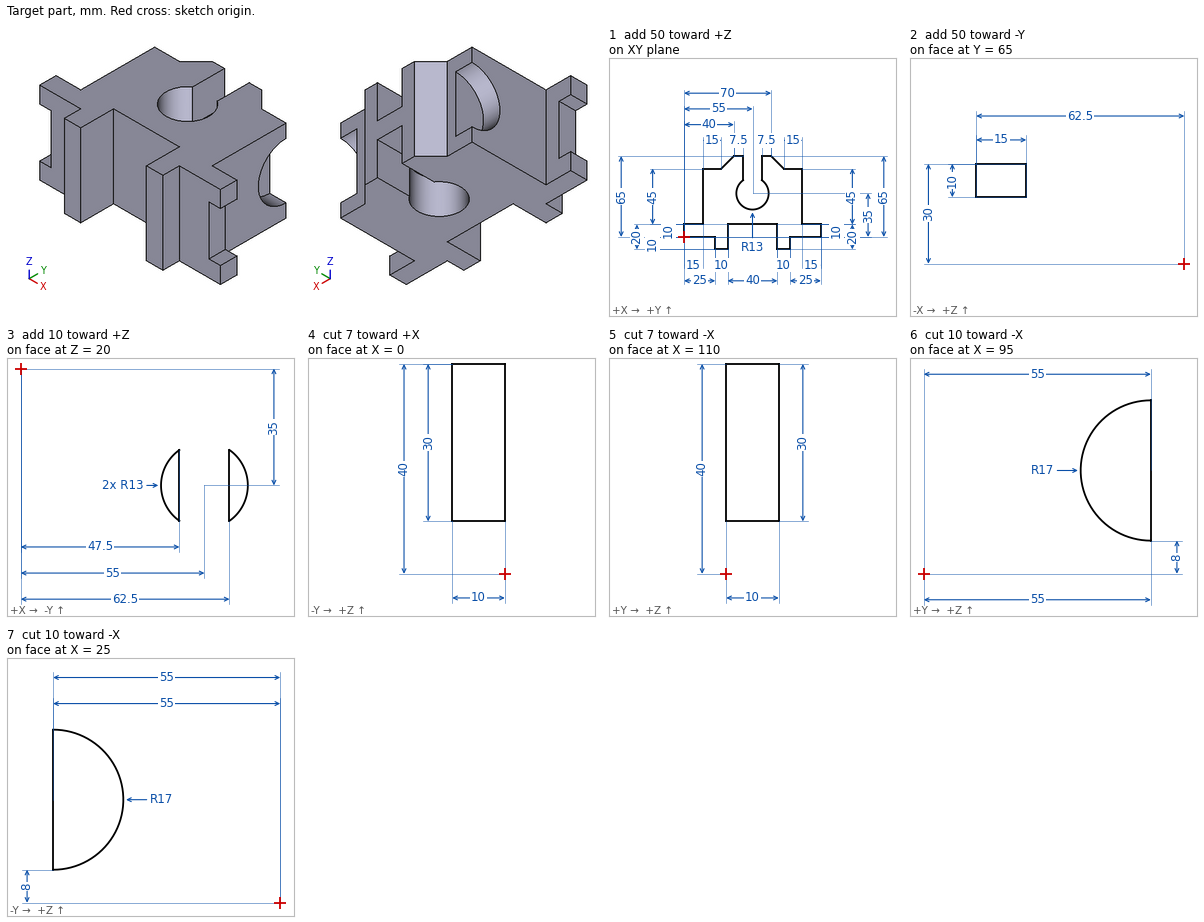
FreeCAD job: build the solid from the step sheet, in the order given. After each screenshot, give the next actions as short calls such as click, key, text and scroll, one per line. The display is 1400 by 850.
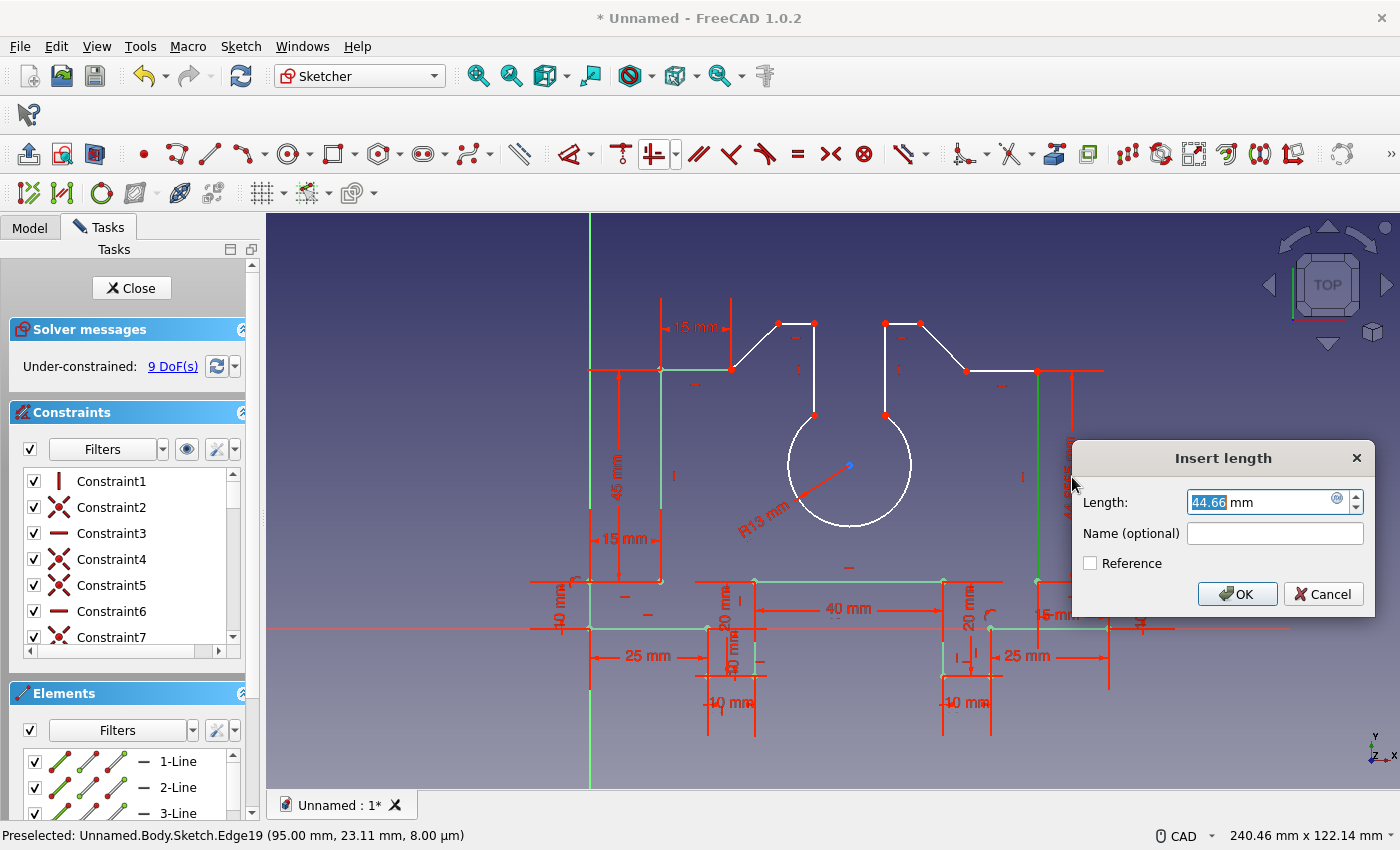
text(45)
key(Return)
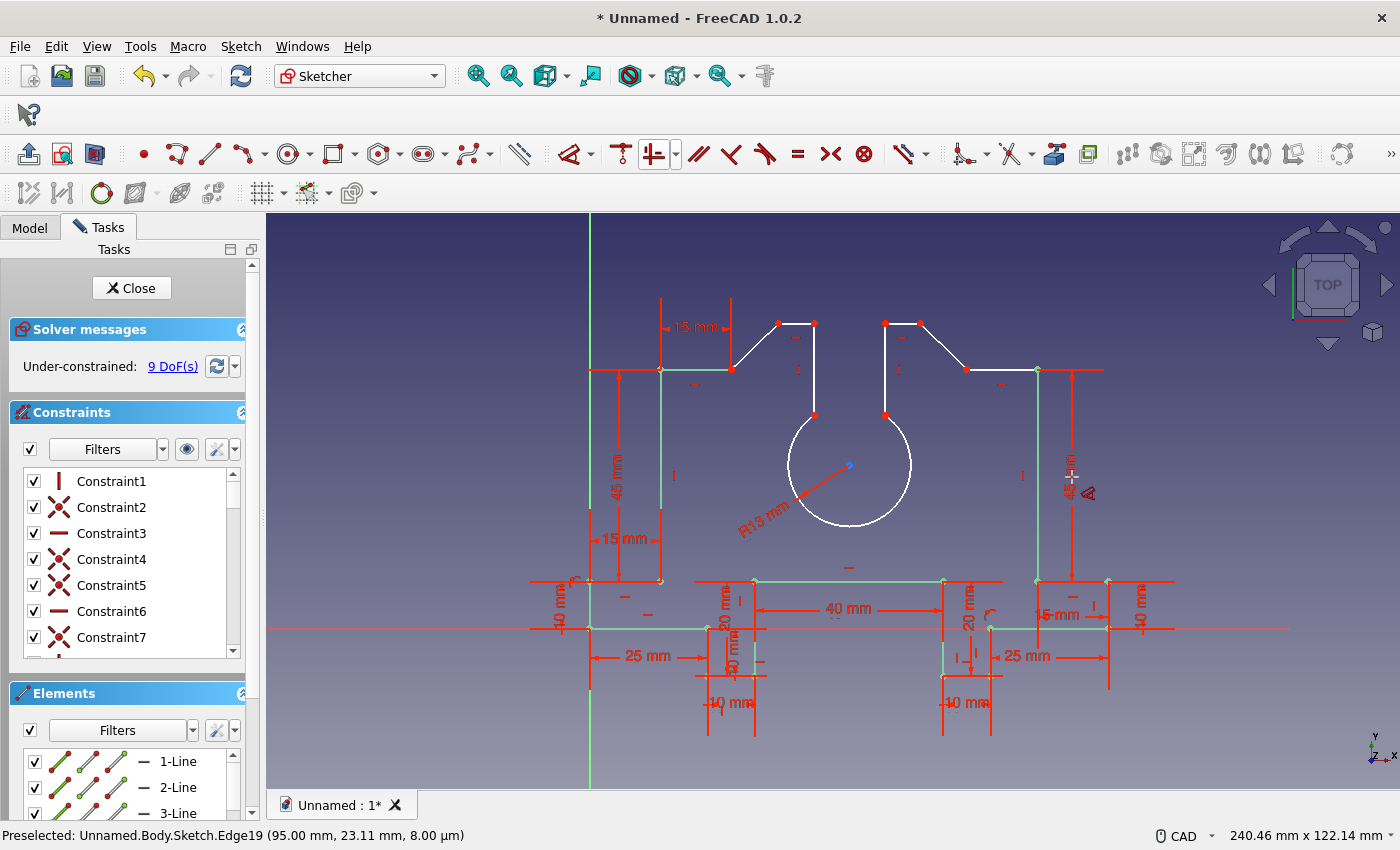
click(1017, 370)
click(1002, 336)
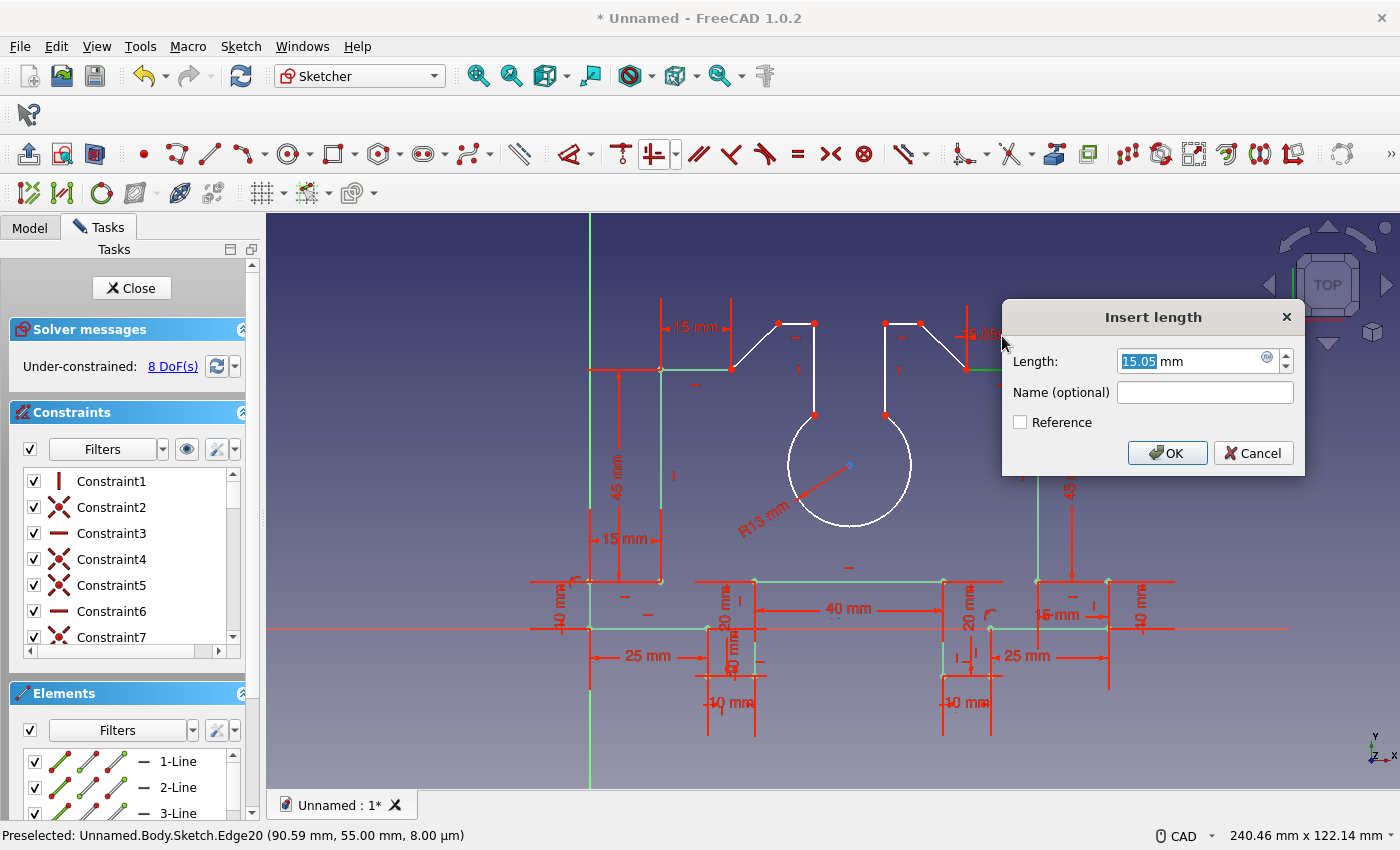
text(15)
key(Return)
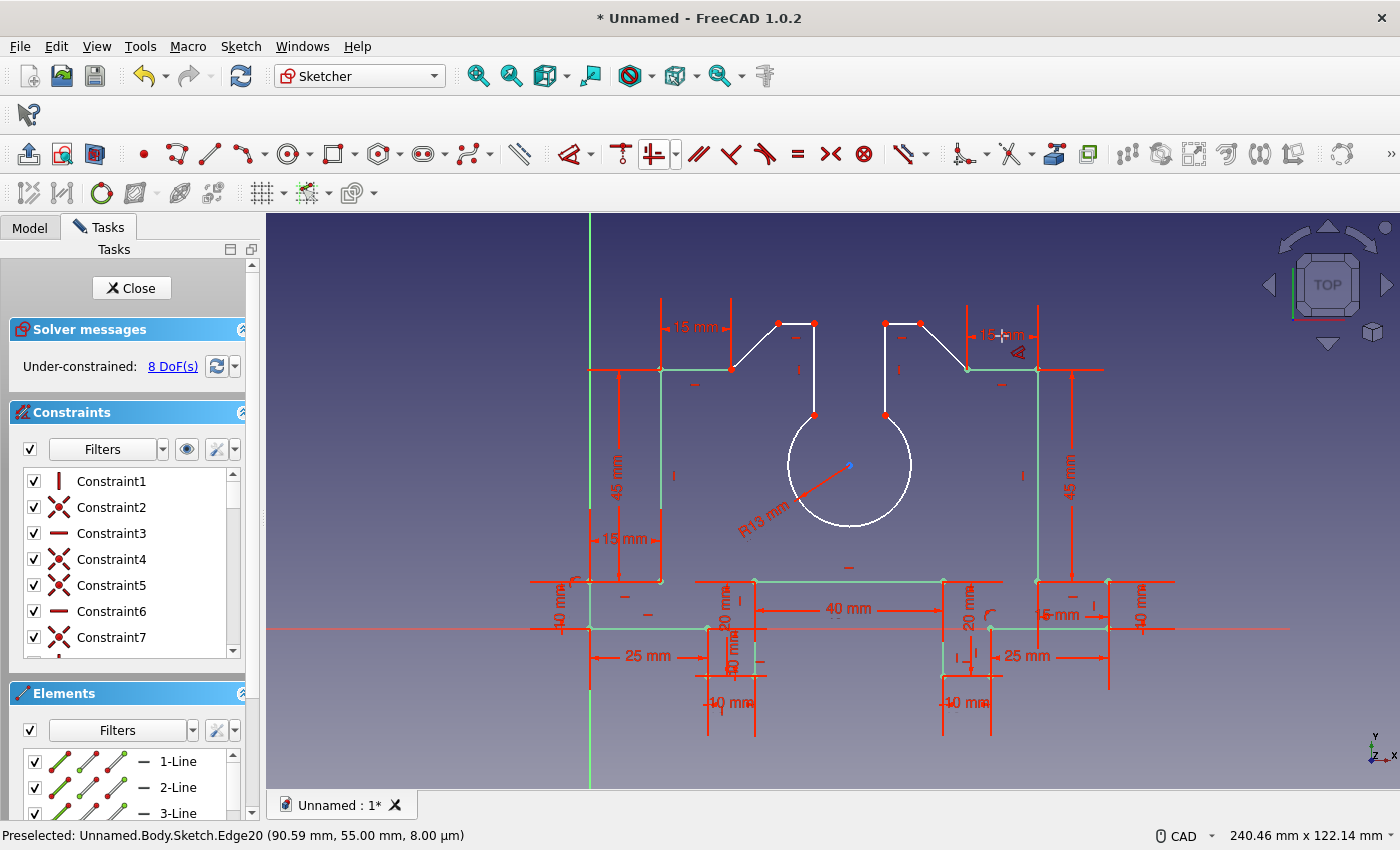
scroll(804, 324, up, 2)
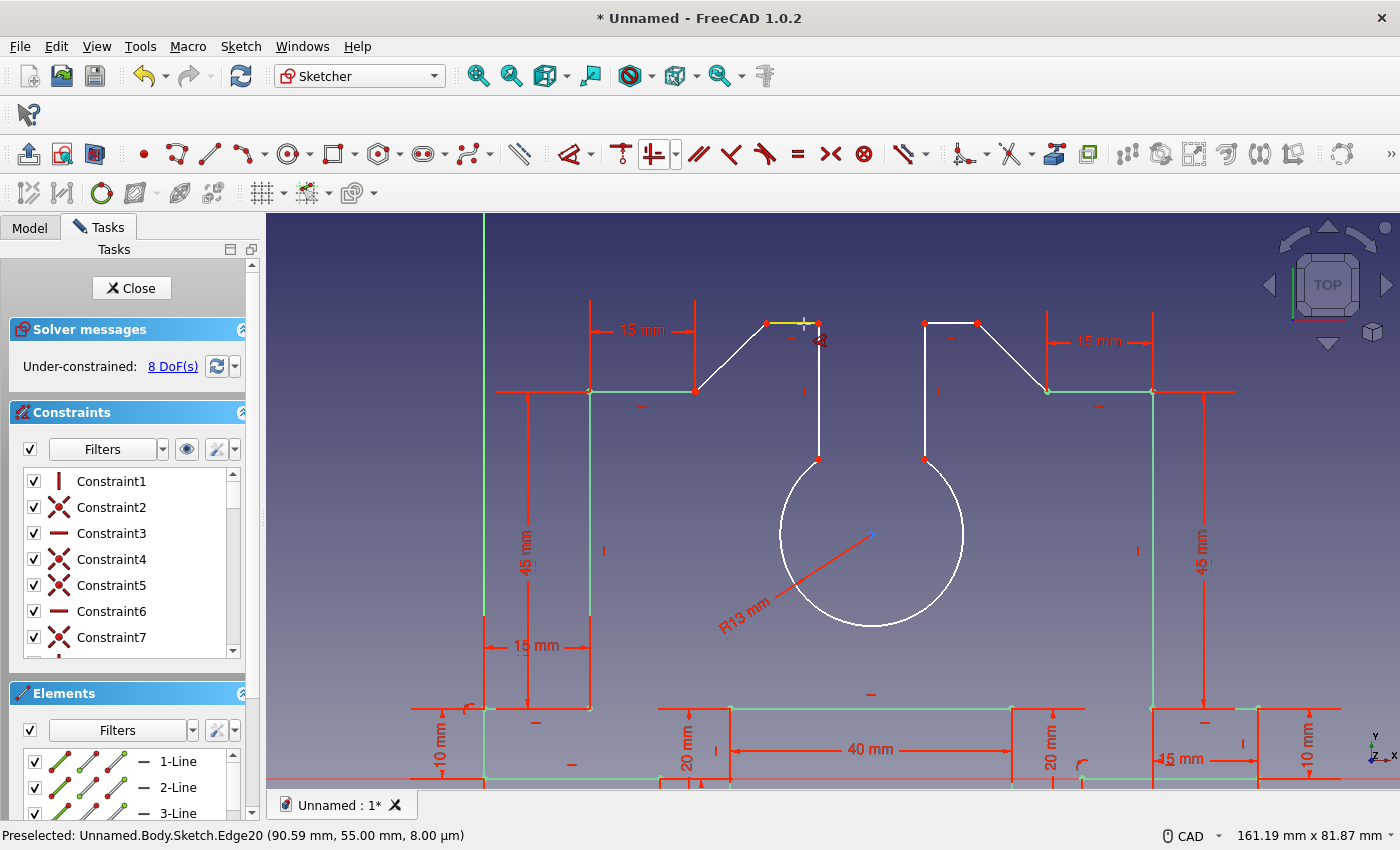
click(803, 323)
click(793, 289)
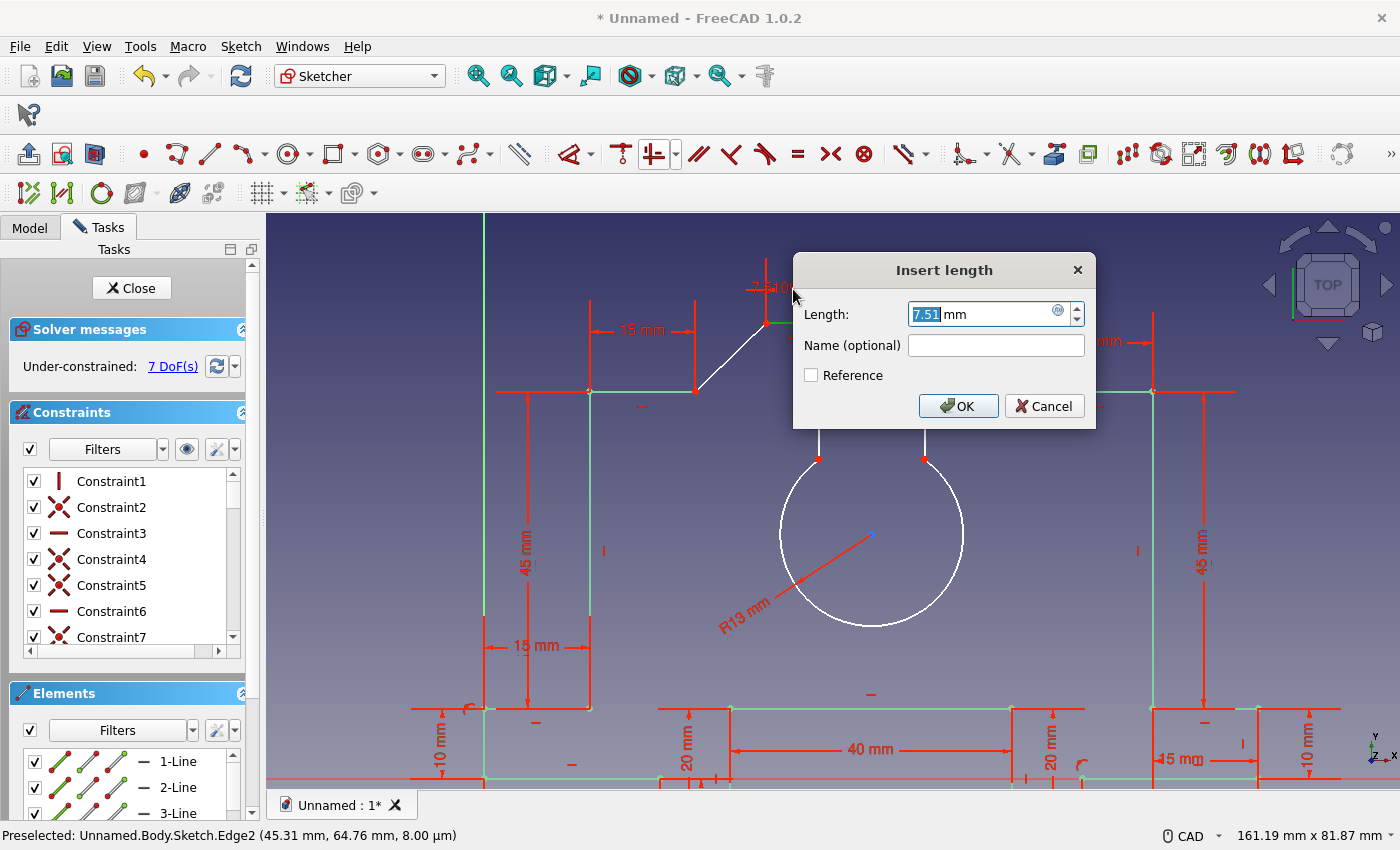
text(7.5)
key(Return)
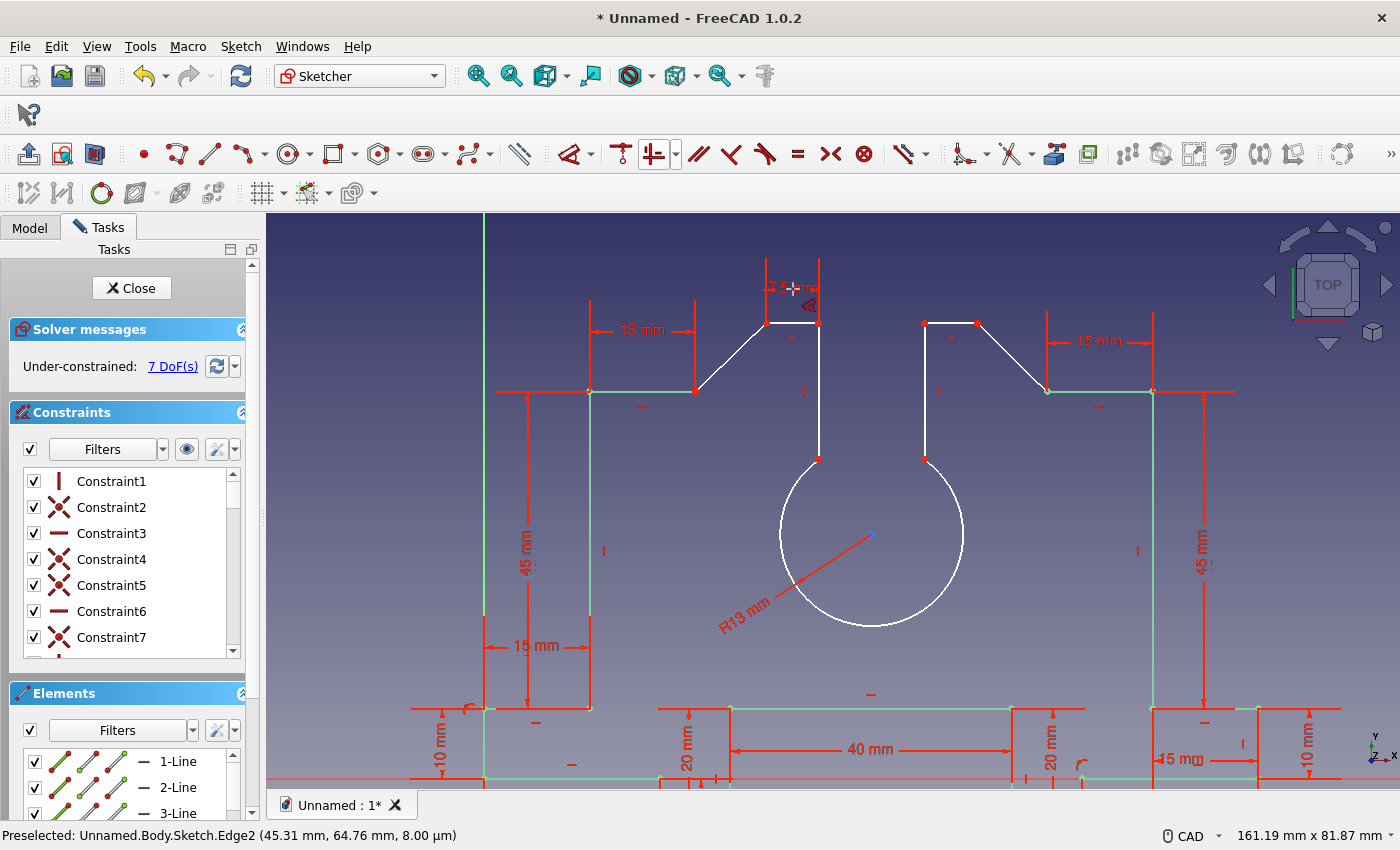
click(962, 323)
click(951, 289)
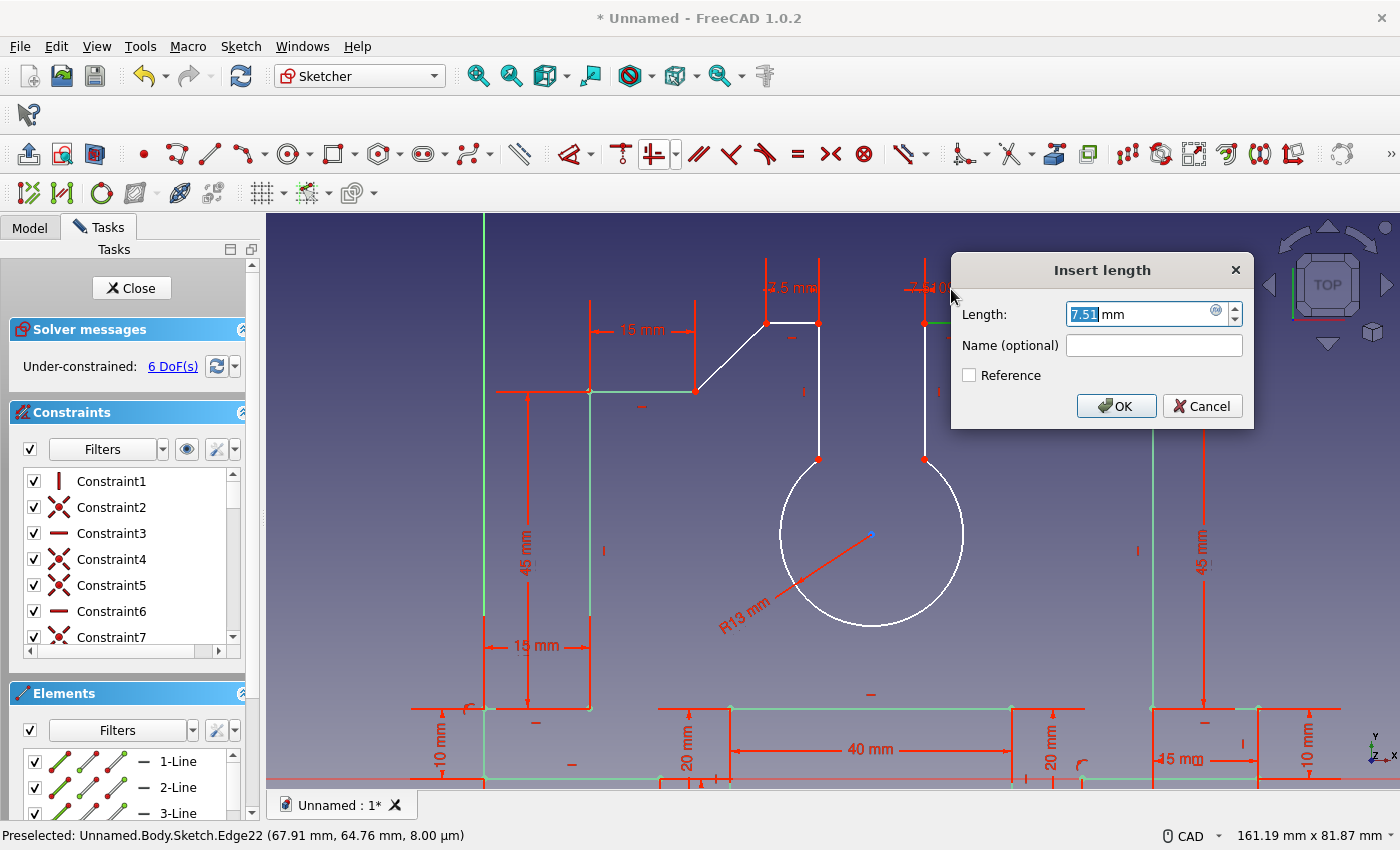
text(7.5)
key(Return)